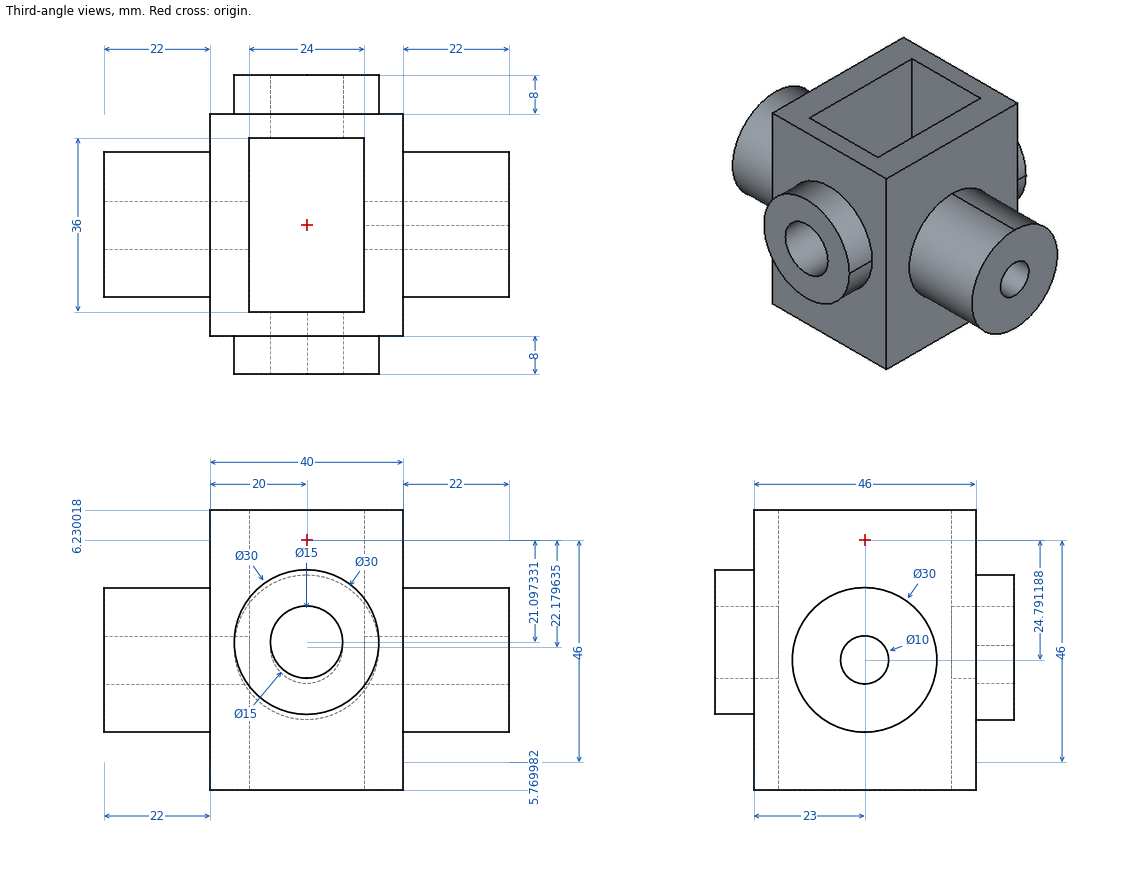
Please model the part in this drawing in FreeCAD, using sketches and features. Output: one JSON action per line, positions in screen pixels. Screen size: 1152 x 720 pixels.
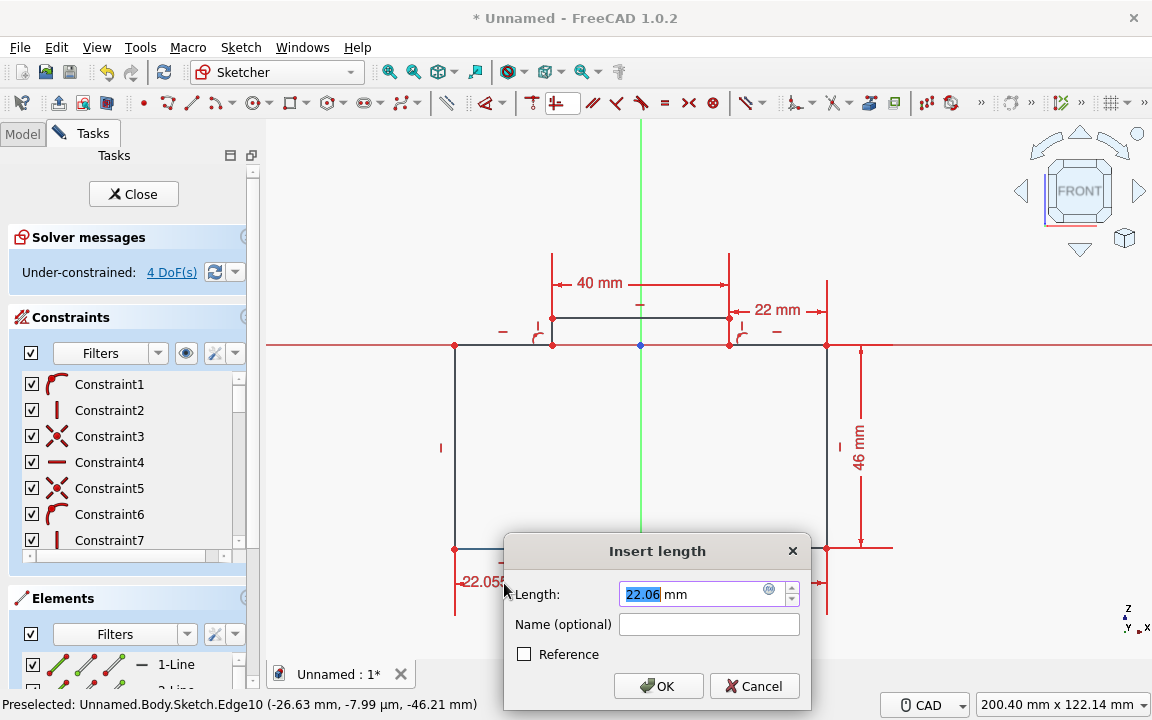
{"action": "type", "text": "22"}
{"action": "key", "text": "Return"}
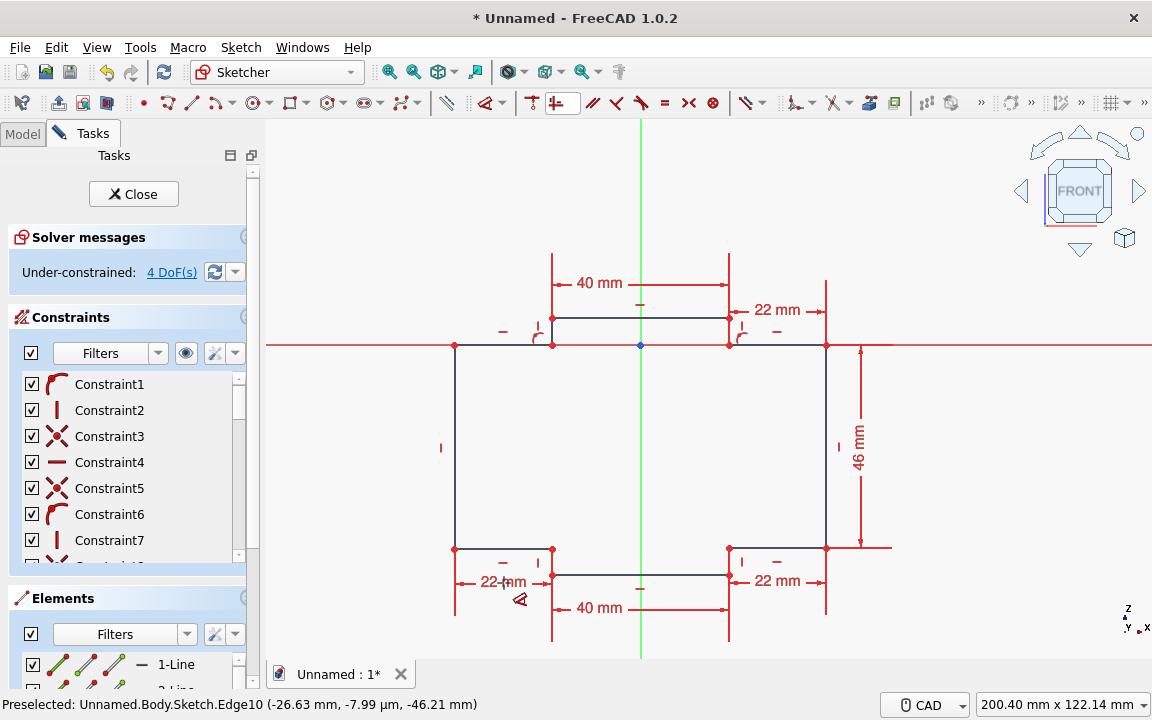
{"action": "left_click", "coordinate": [455, 488]}
{"action": "left_click", "coordinate": [421, 447]}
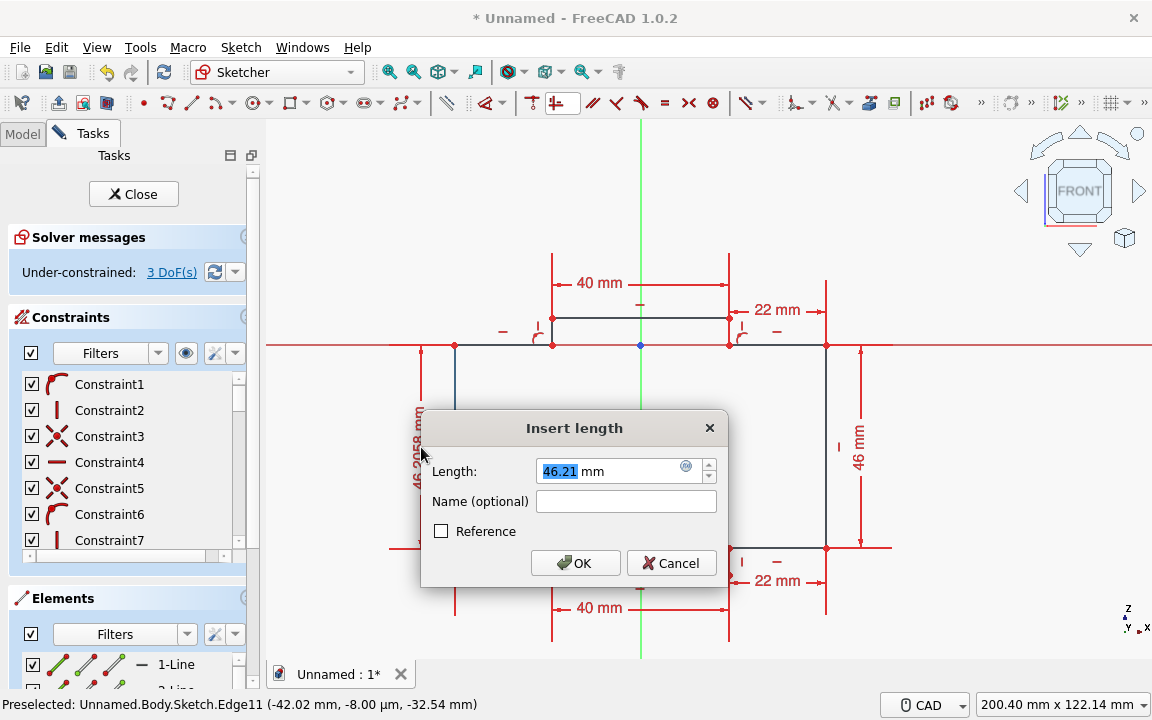
{"action": "type", "text": "46"}
{"action": "key", "text": "Return"}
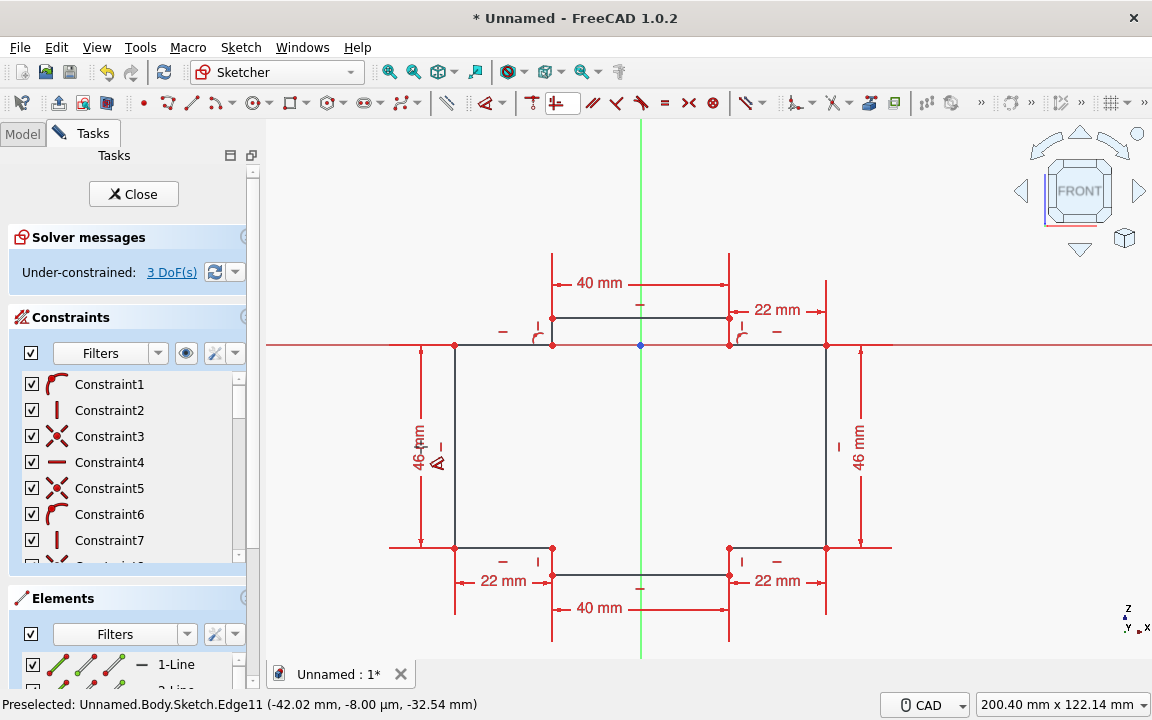
{"action": "left_click", "coordinate": [552, 345]}
{"action": "left_click", "coordinate": [596, 379]}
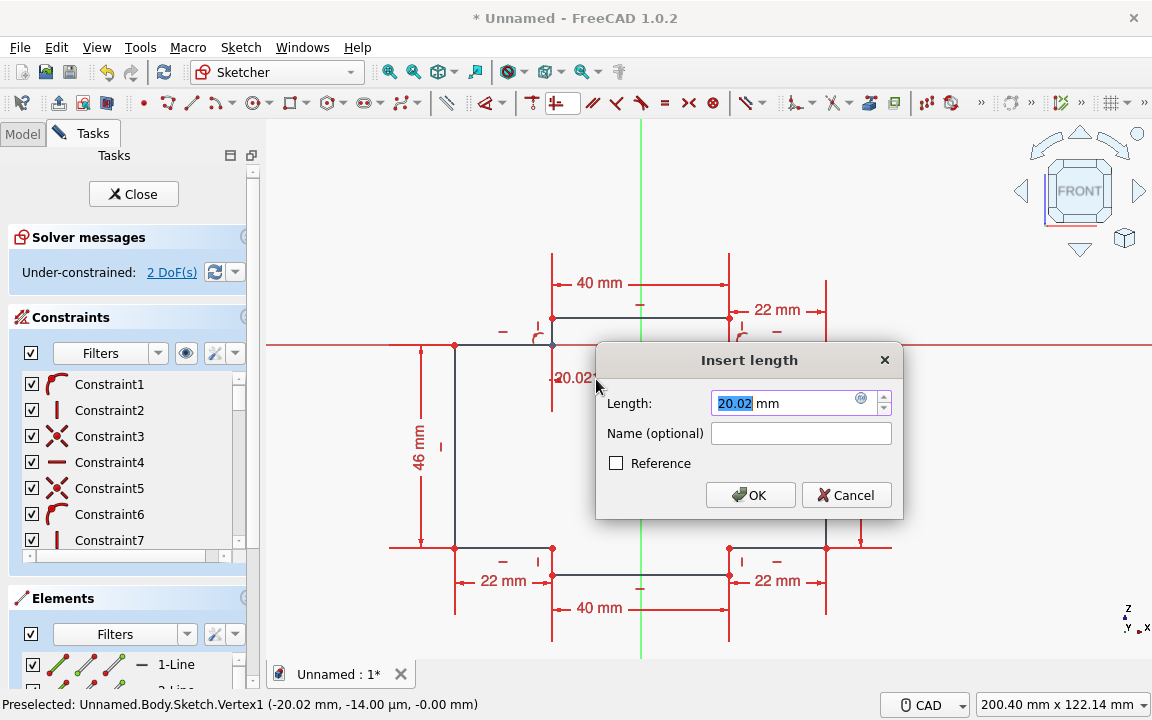
{"action": "type", "text": "20"}
{"action": "key", "text": "Return"}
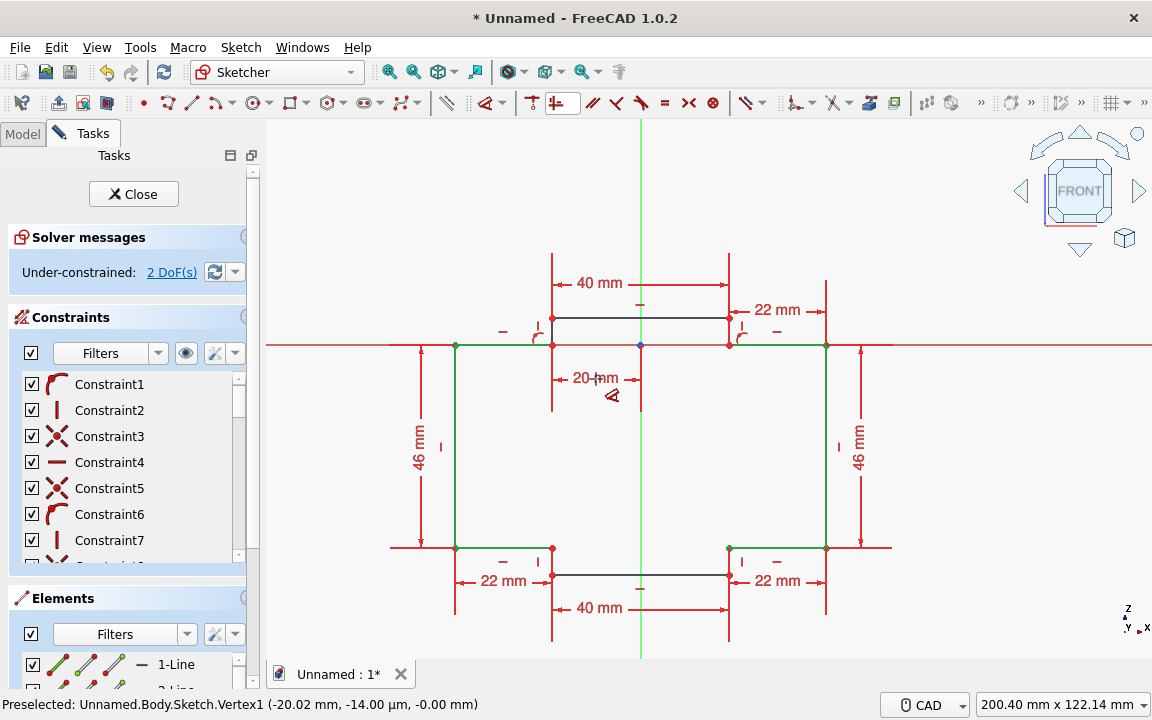
{"action": "scroll", "coordinate": [552, 334], "scroll_direction": "up", "scroll_amount": 2}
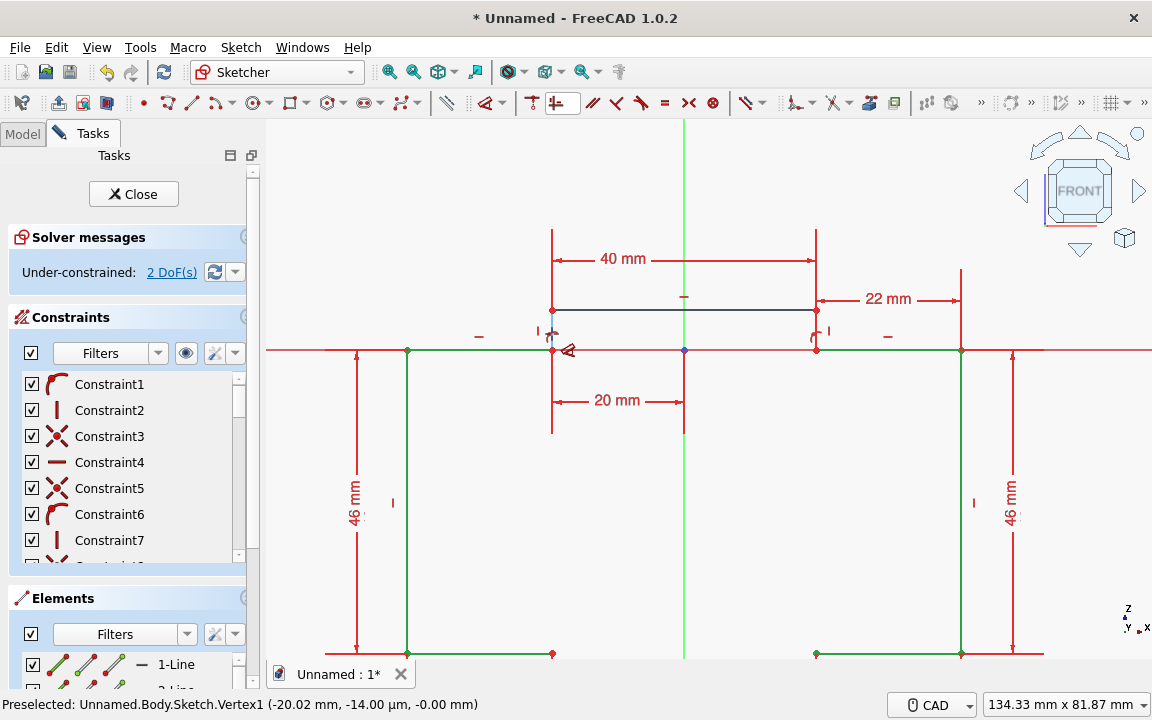
{"action": "left_click", "coordinate": [552, 334]}
{"action": "left_click", "coordinate": [518, 330]}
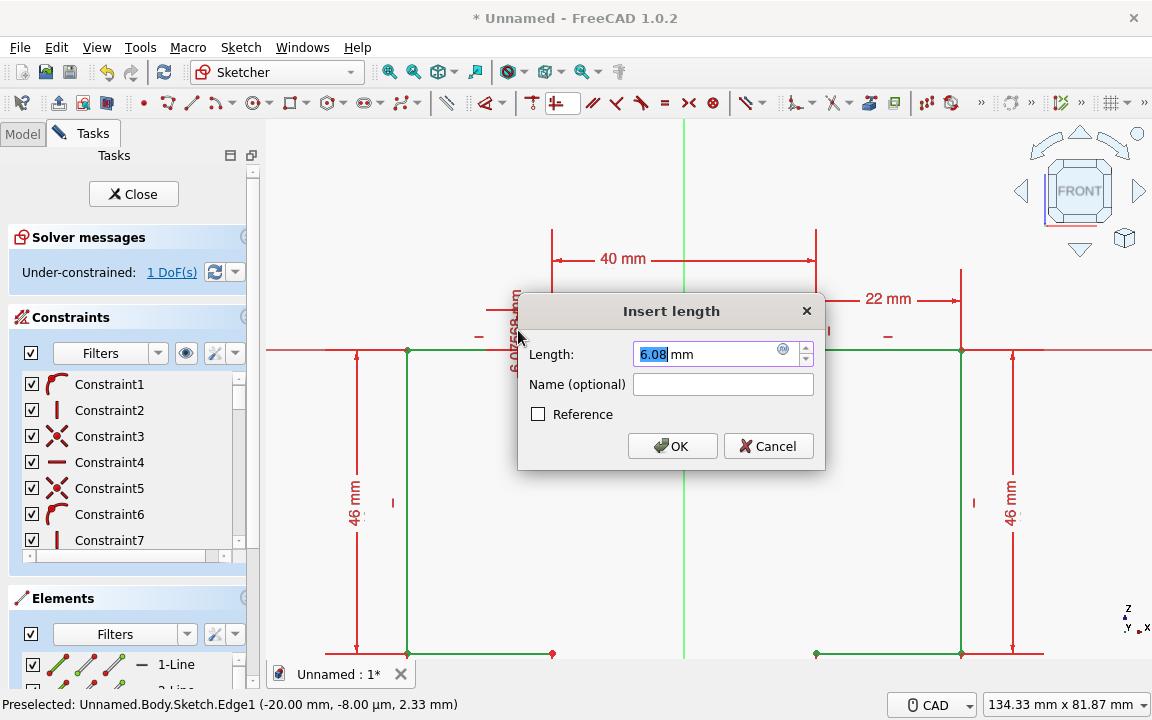
{"action": "type", "text": "6.230018"}
{"action": "key", "text": "Return"}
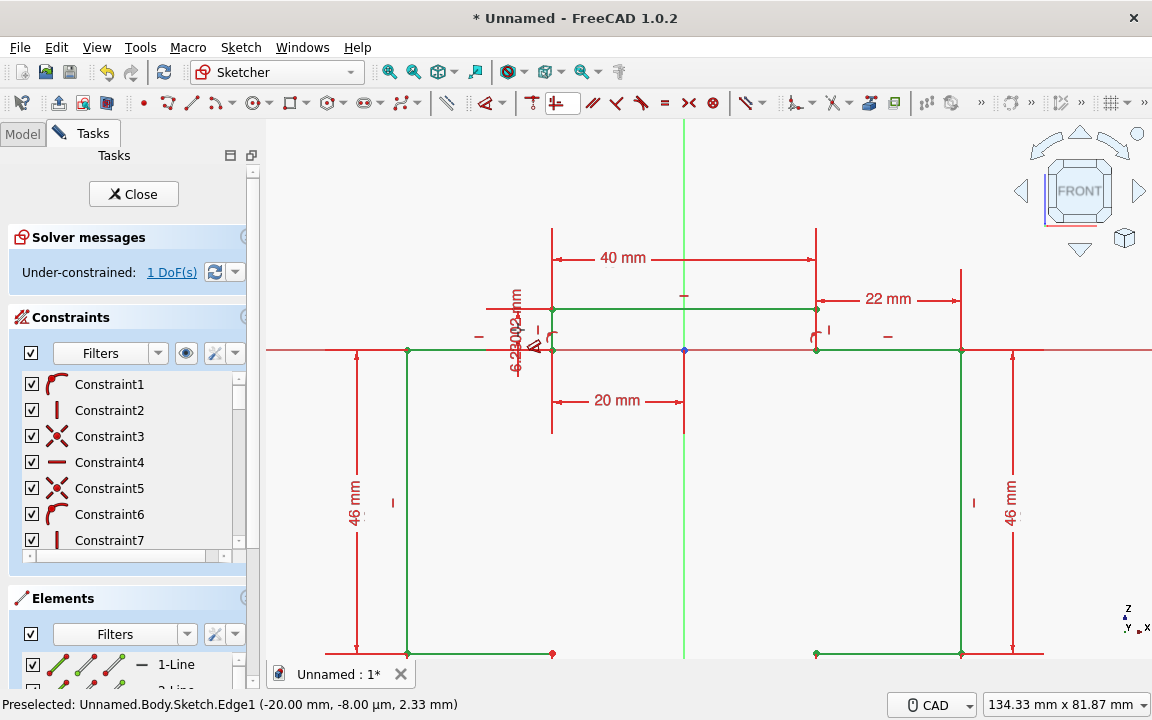
{"action": "scroll", "coordinate": [443, 147], "scroll_direction": "down", "scroll_amount": 1}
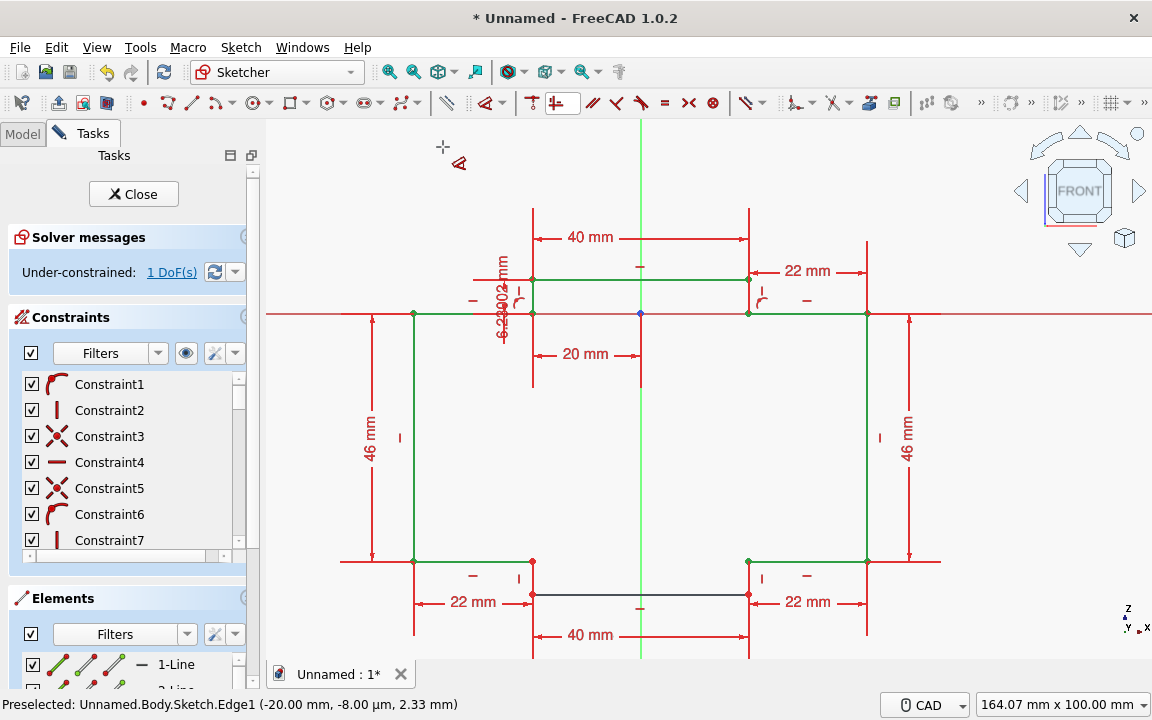
{"action": "scroll", "coordinate": [749, 572], "scroll_direction": "up", "scroll_amount": 2}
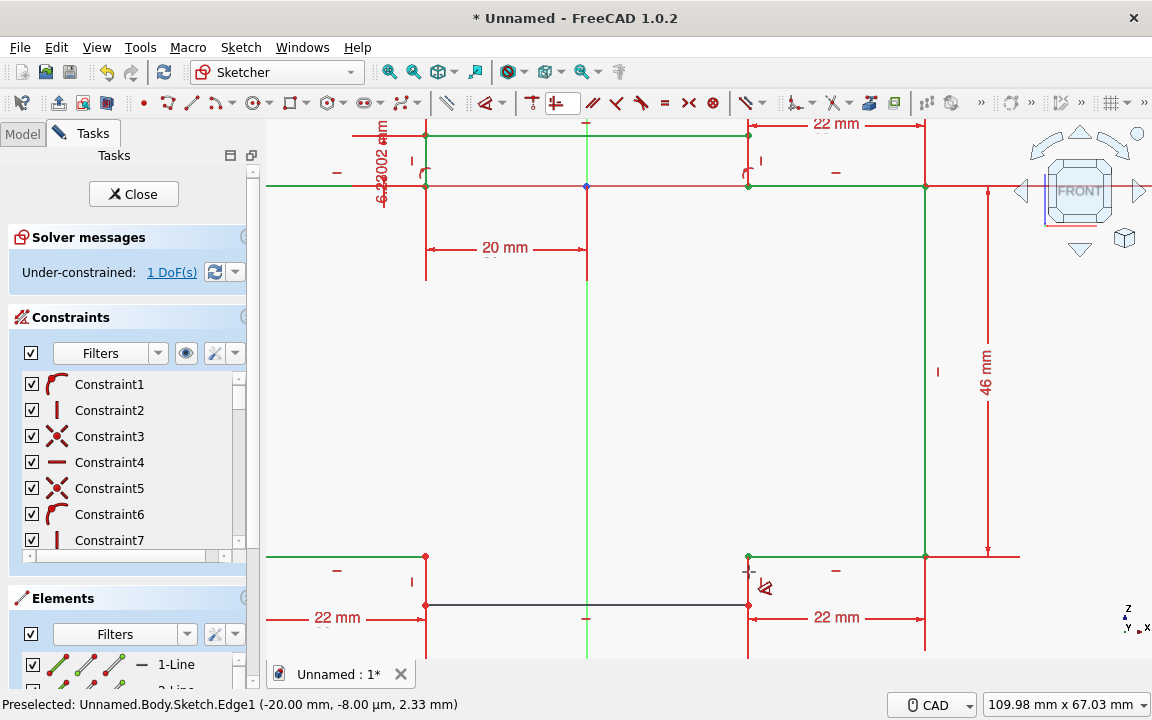
{"action": "left_click", "coordinate": [748, 571]}
{"action": "left_click", "coordinate": [782, 581]}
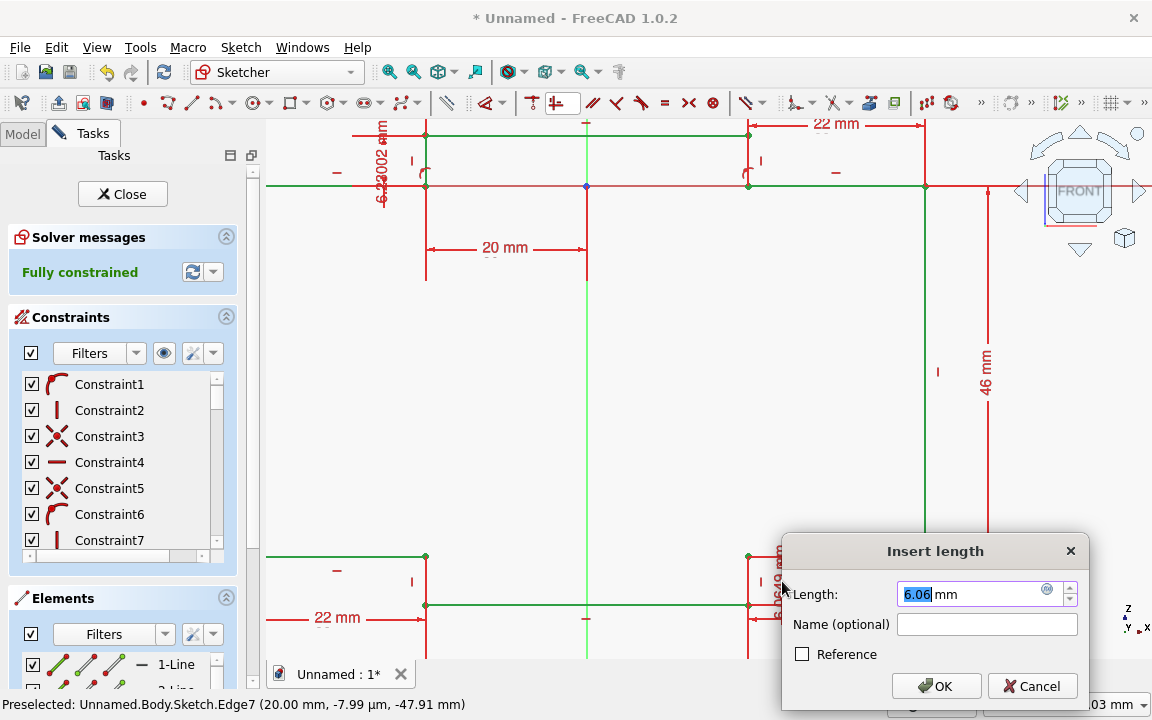
{"action": "type", "text": "5.769982"}
{"action": "key", "text": "Return"}
{"action": "key", "text": "Escape"}